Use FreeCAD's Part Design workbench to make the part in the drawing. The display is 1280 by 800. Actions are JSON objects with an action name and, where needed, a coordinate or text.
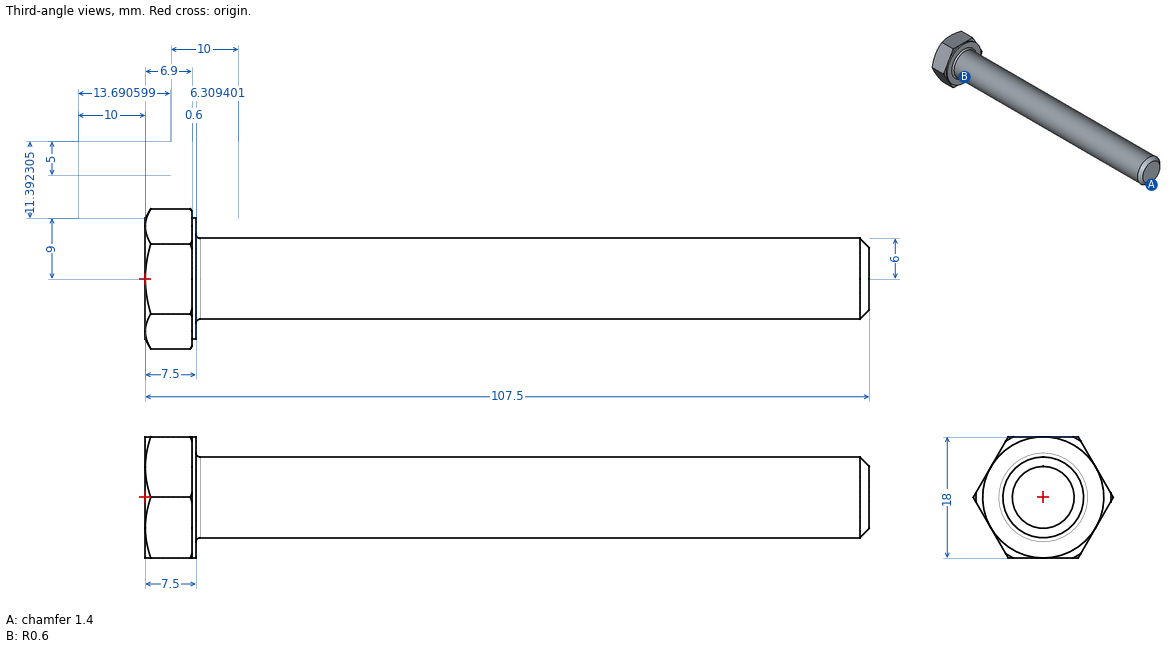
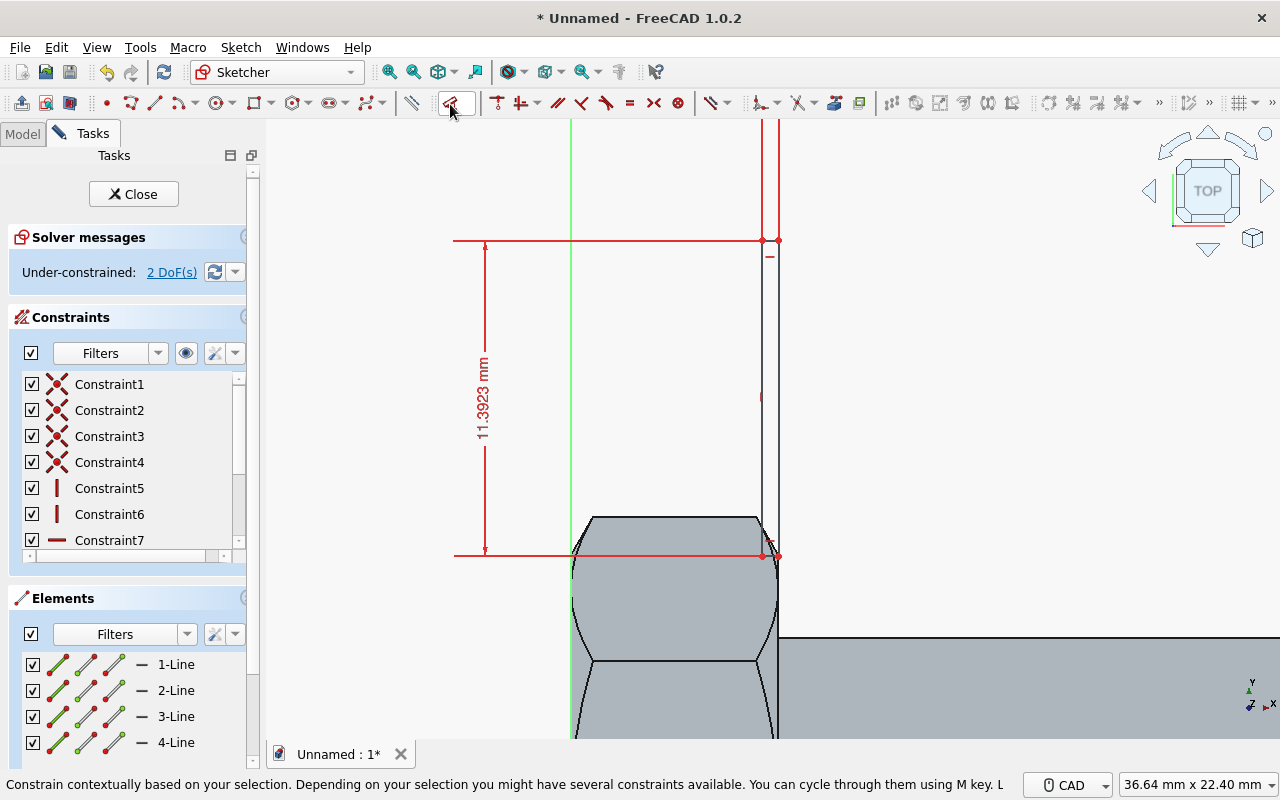
{"action": "left_click", "coordinate": [762, 556]}
{"action": "left_click", "coordinate": [537, 634]}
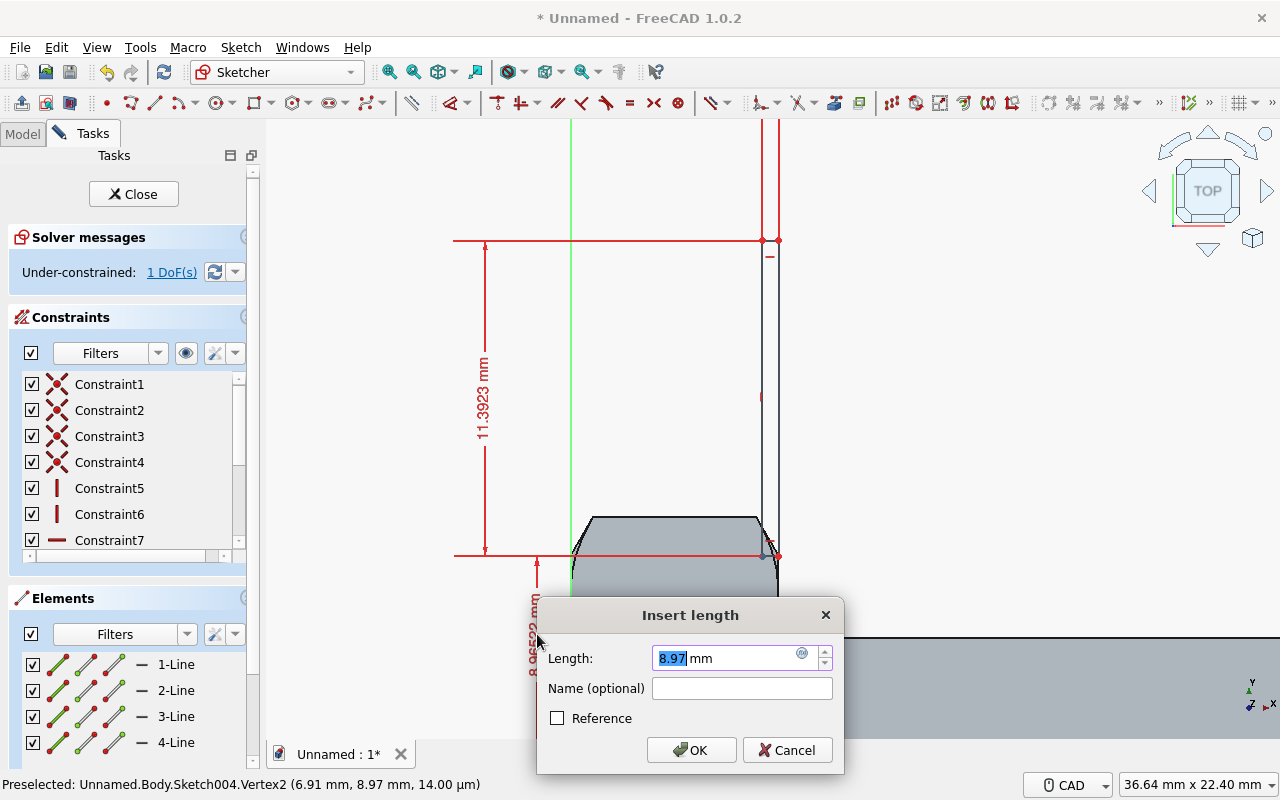
{"action": "type", "text": "9"}
{"action": "key", "text": "Return"}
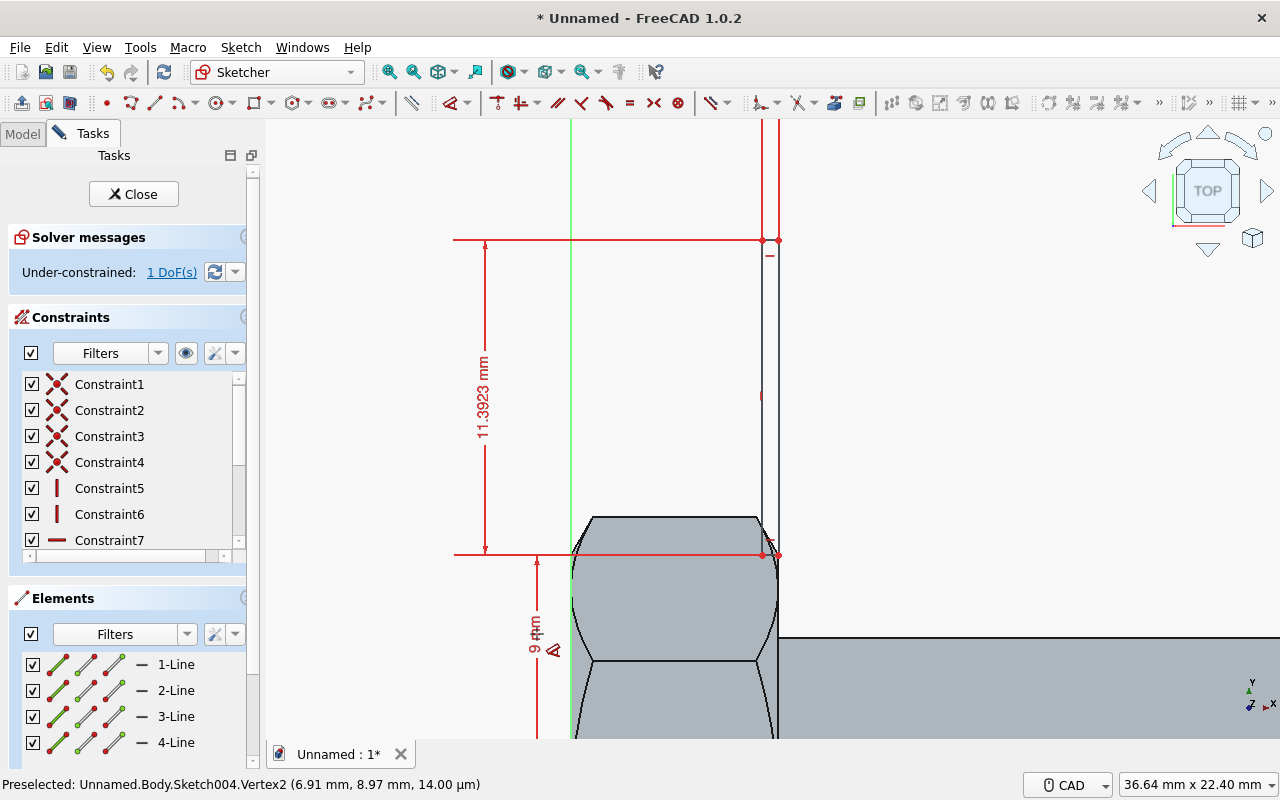
{"action": "left_click", "coordinate": [762, 240]}
{"action": "left_click", "coordinate": [666, 206]}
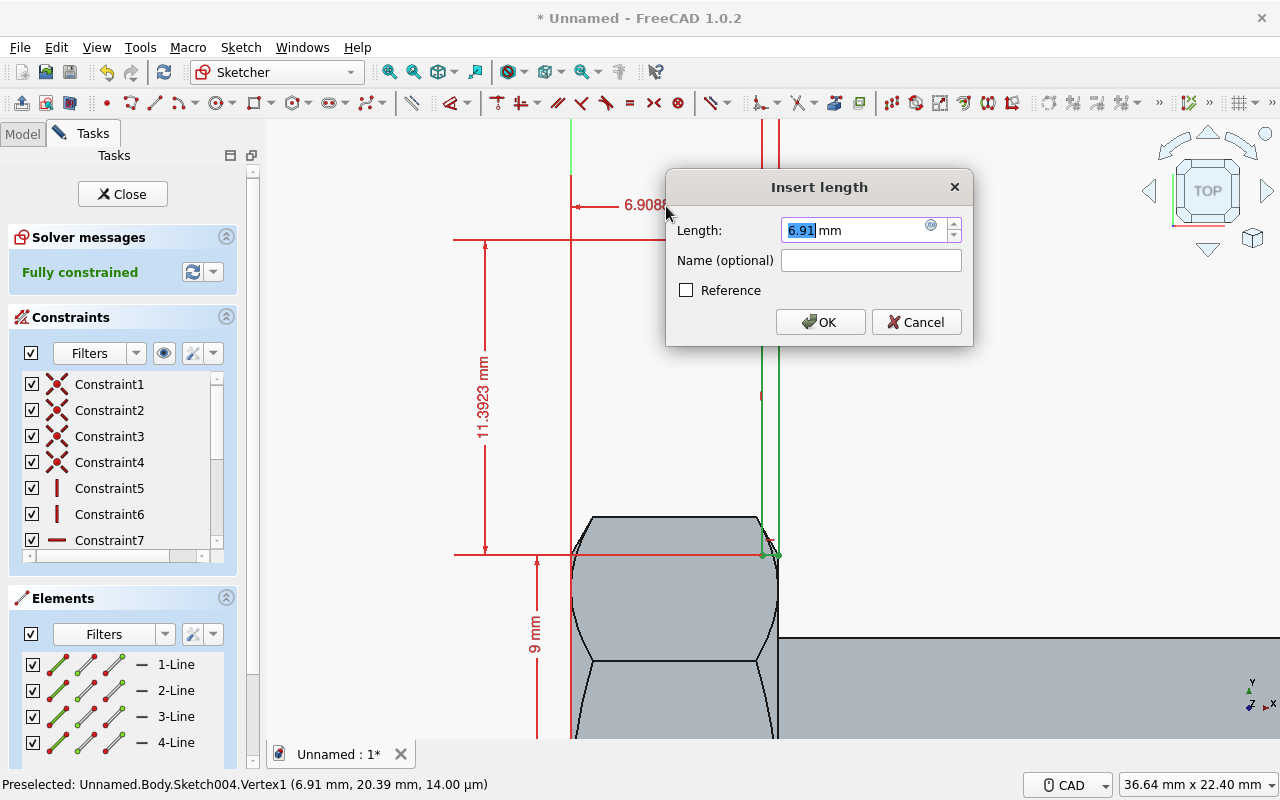
{"action": "type", "text": "6.9"}
{"action": "key", "text": "Return"}
{"action": "key", "text": "Escape"}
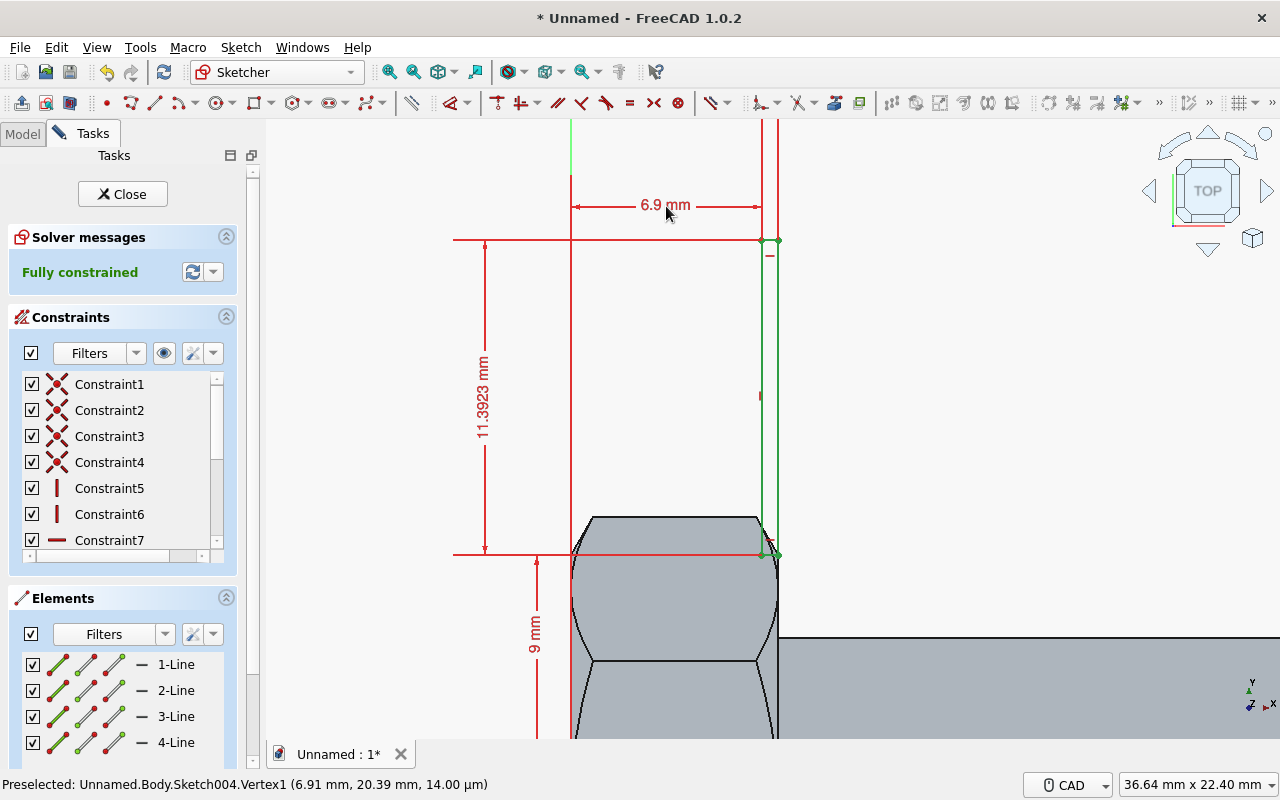
{"action": "left_click", "coordinate": [123, 194]}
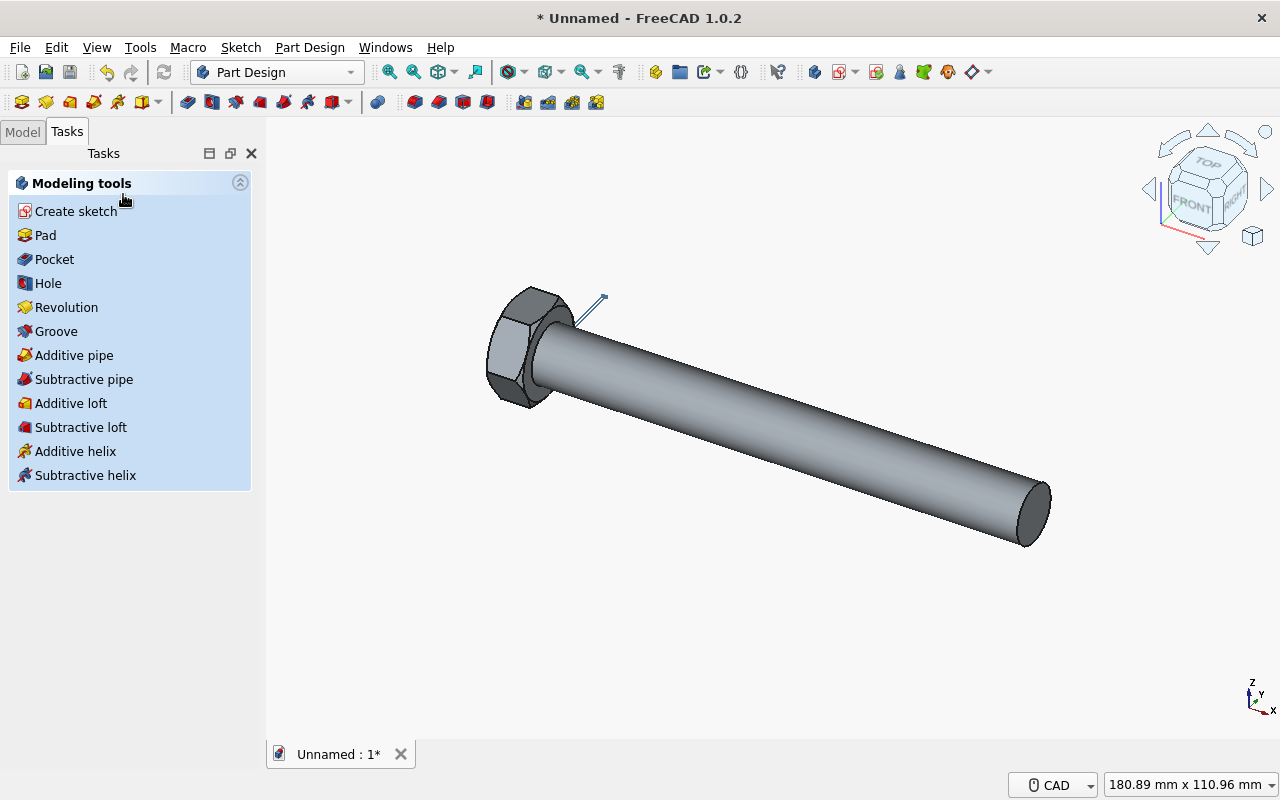
{"action": "left_click", "coordinate": [236, 102]}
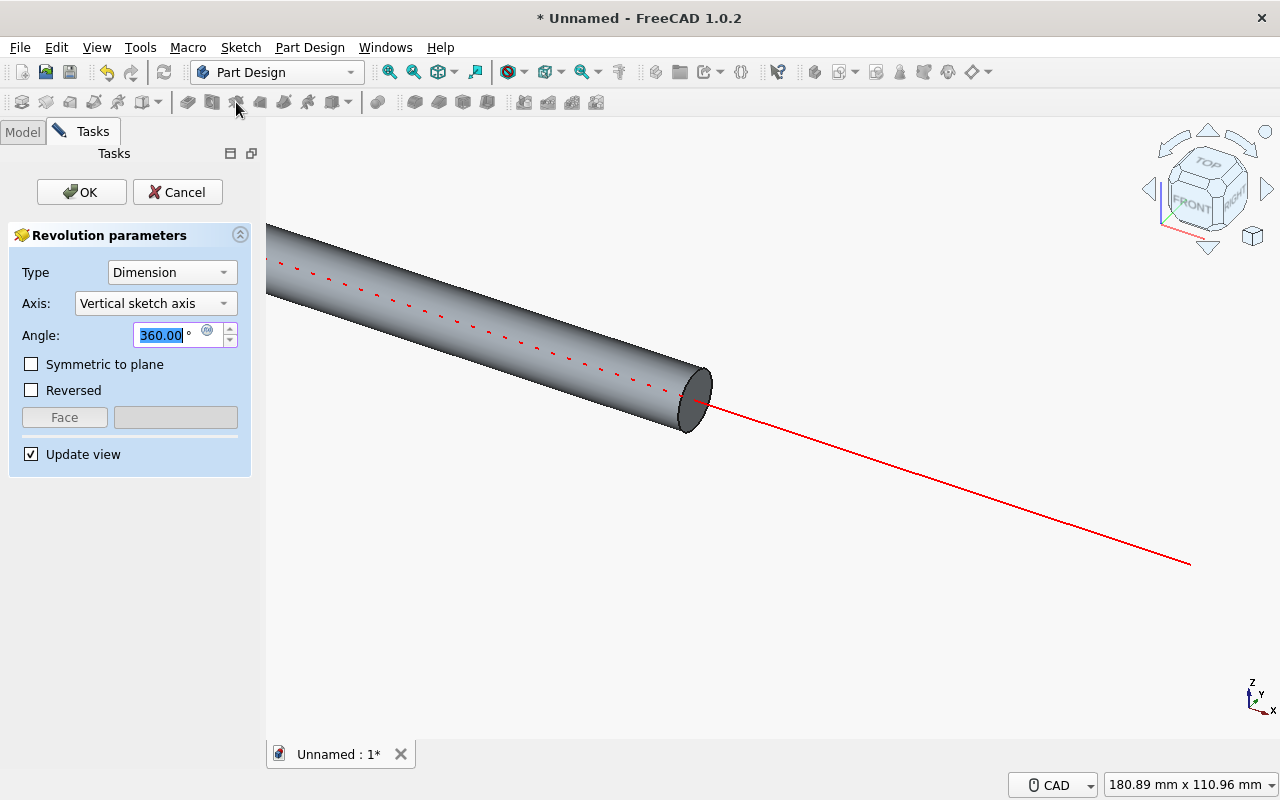
{"action": "left_click", "coordinate": [156, 304]}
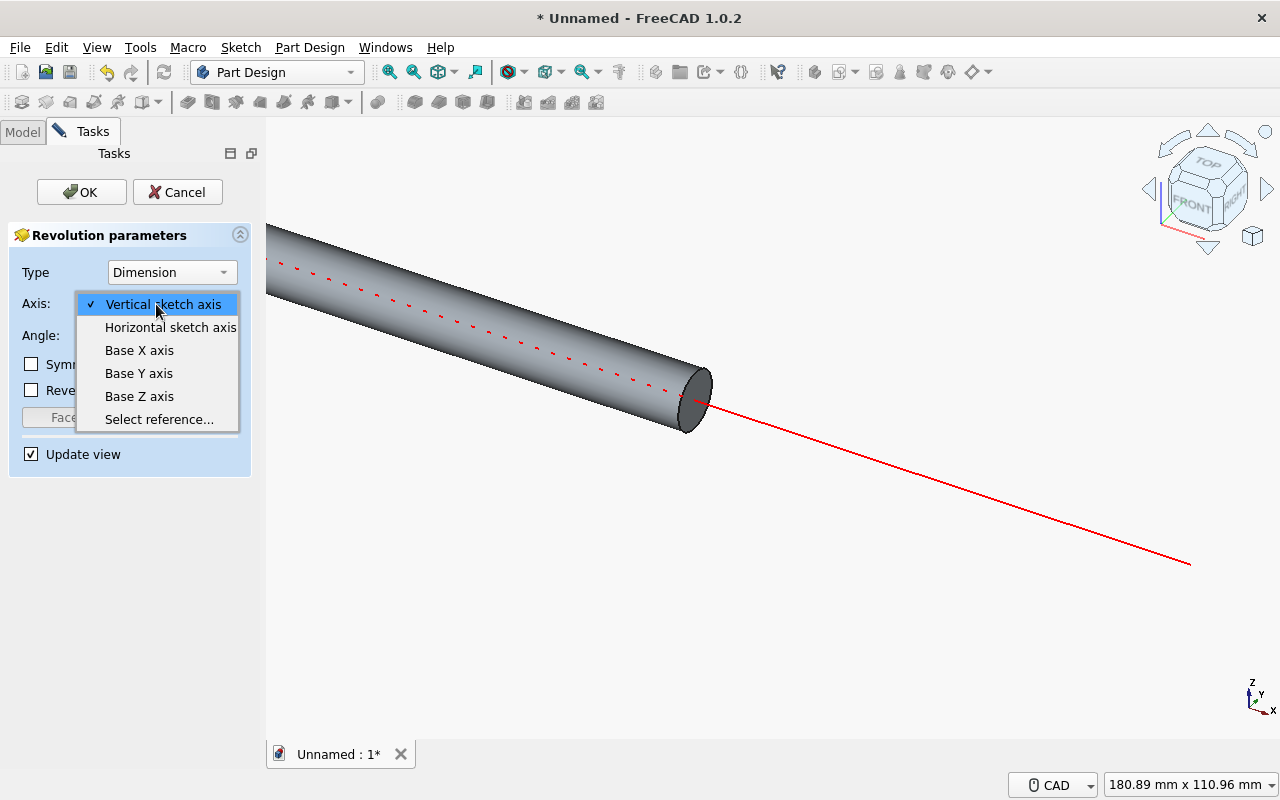
{"action": "left_click", "coordinate": [156, 328]}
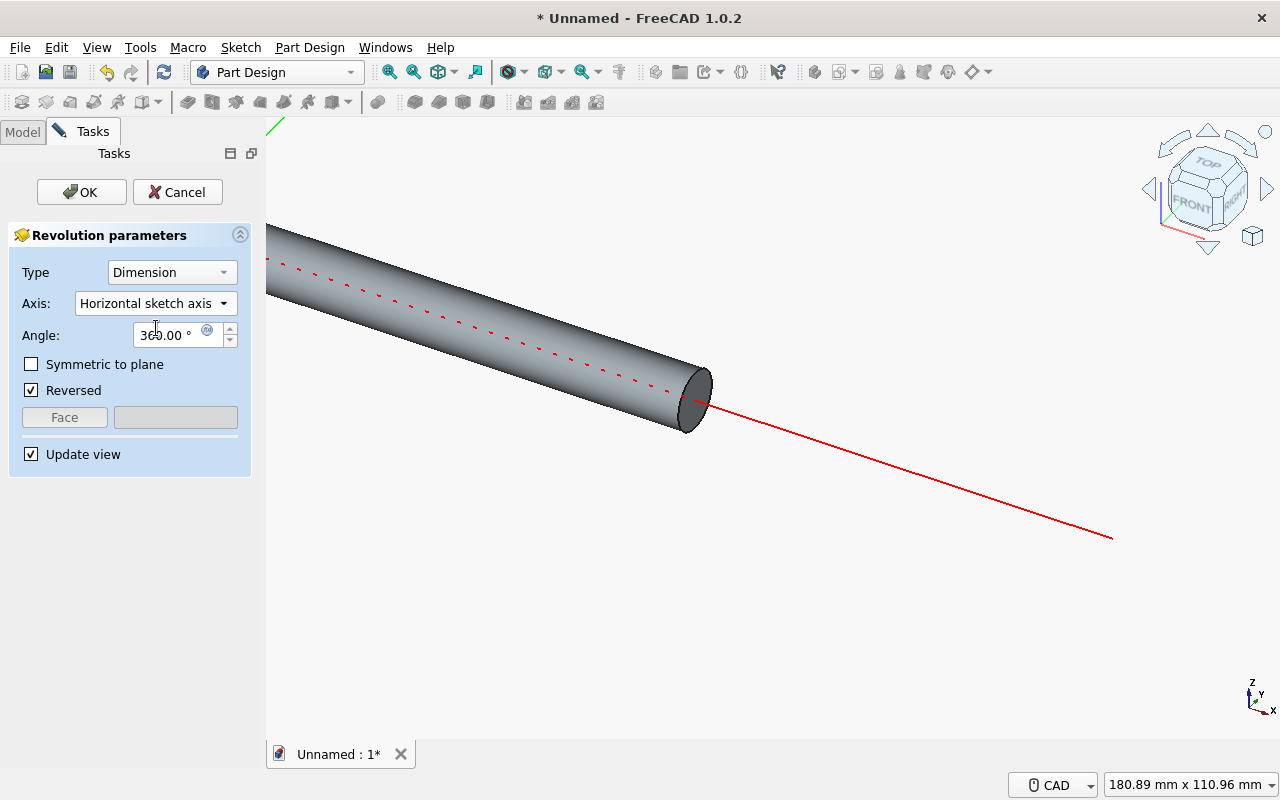
{"action": "left_click", "coordinate": [82, 192]}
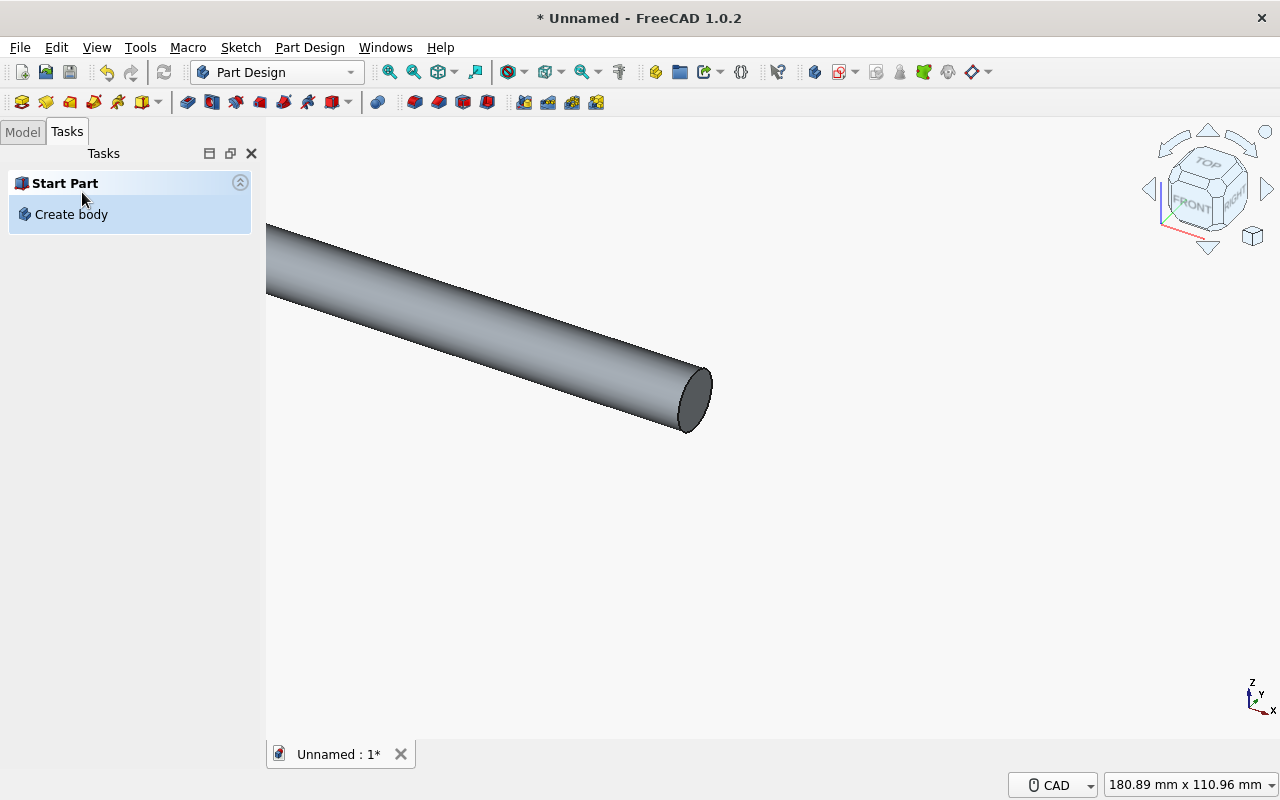
{"action": "key", "text": "v f"}